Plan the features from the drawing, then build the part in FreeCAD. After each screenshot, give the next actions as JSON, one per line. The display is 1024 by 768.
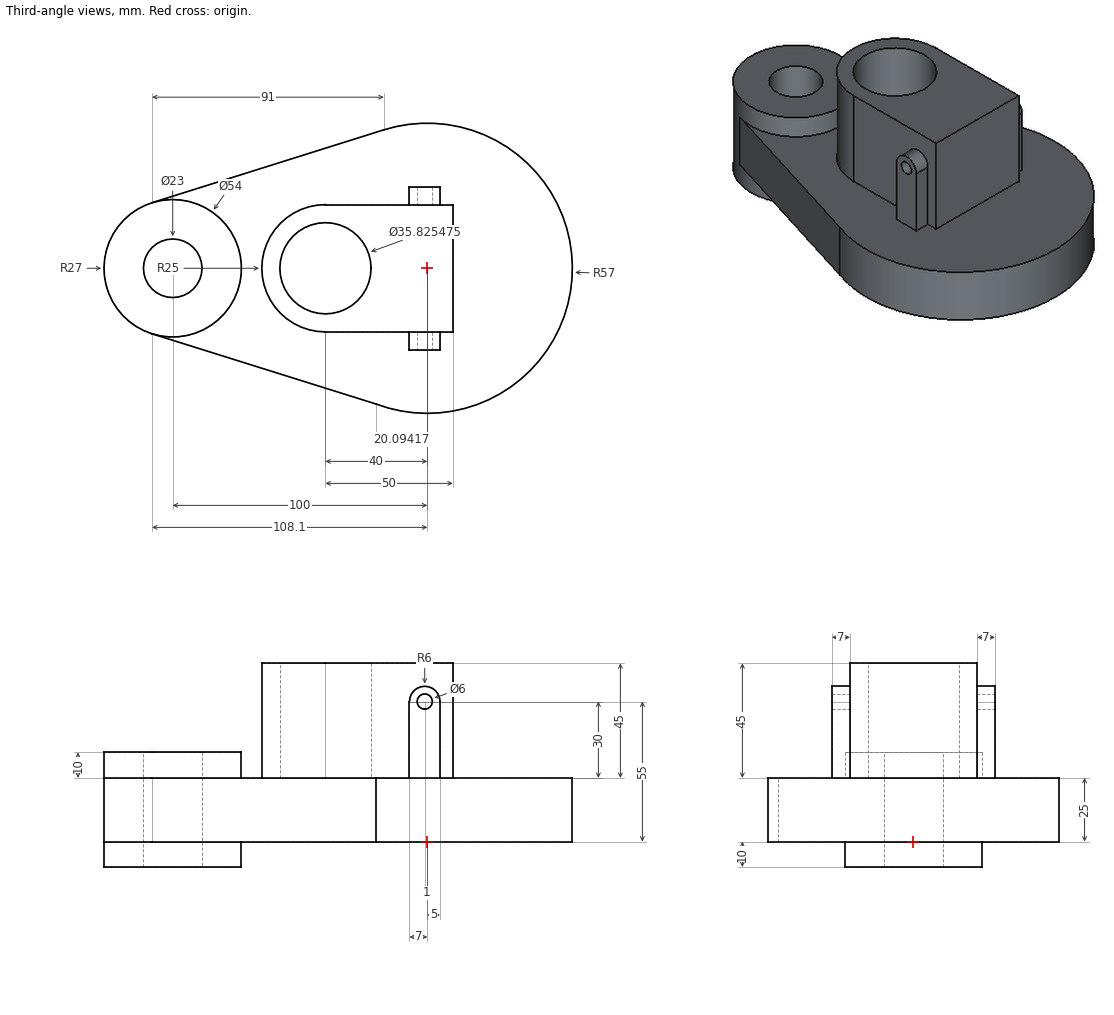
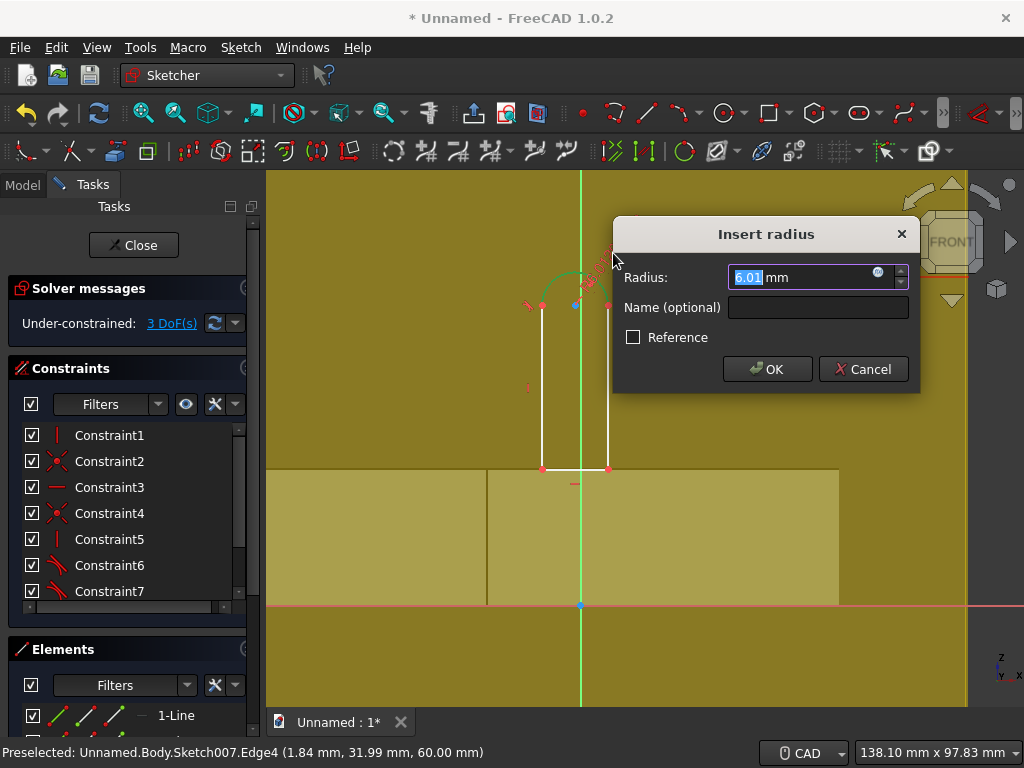
{"action": "type", "text": "6"}
{"action": "key", "text": "Return"}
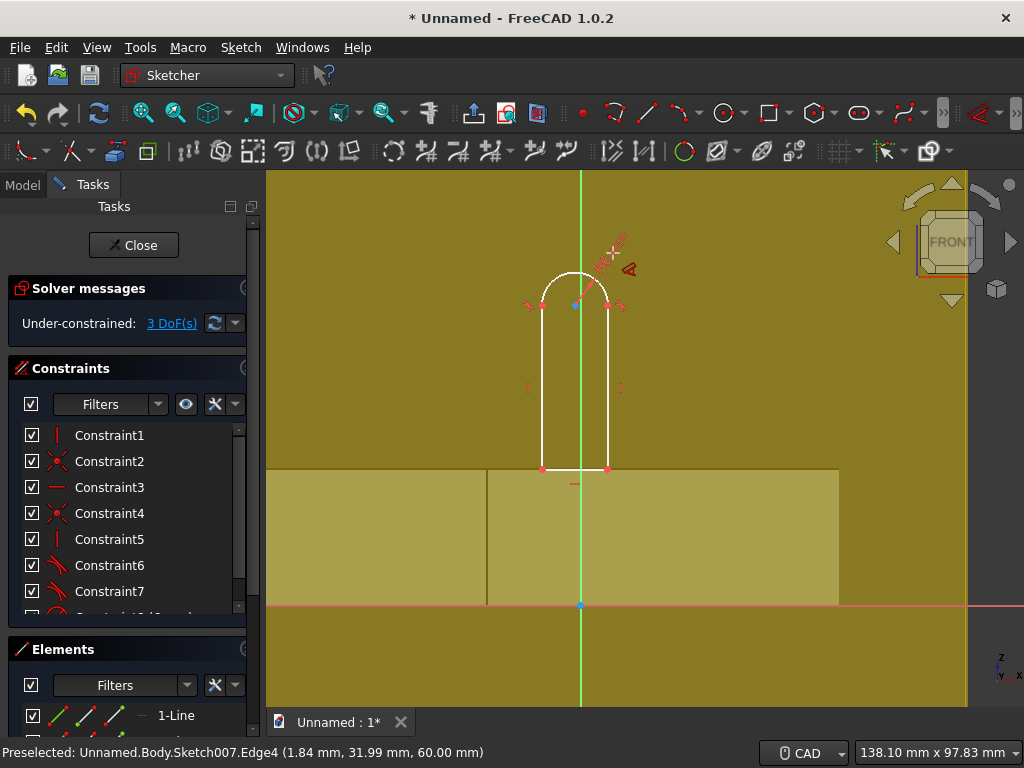
{"action": "left_click", "coordinate": [608, 355]}
{"action": "left_click", "coordinate": [642, 388]}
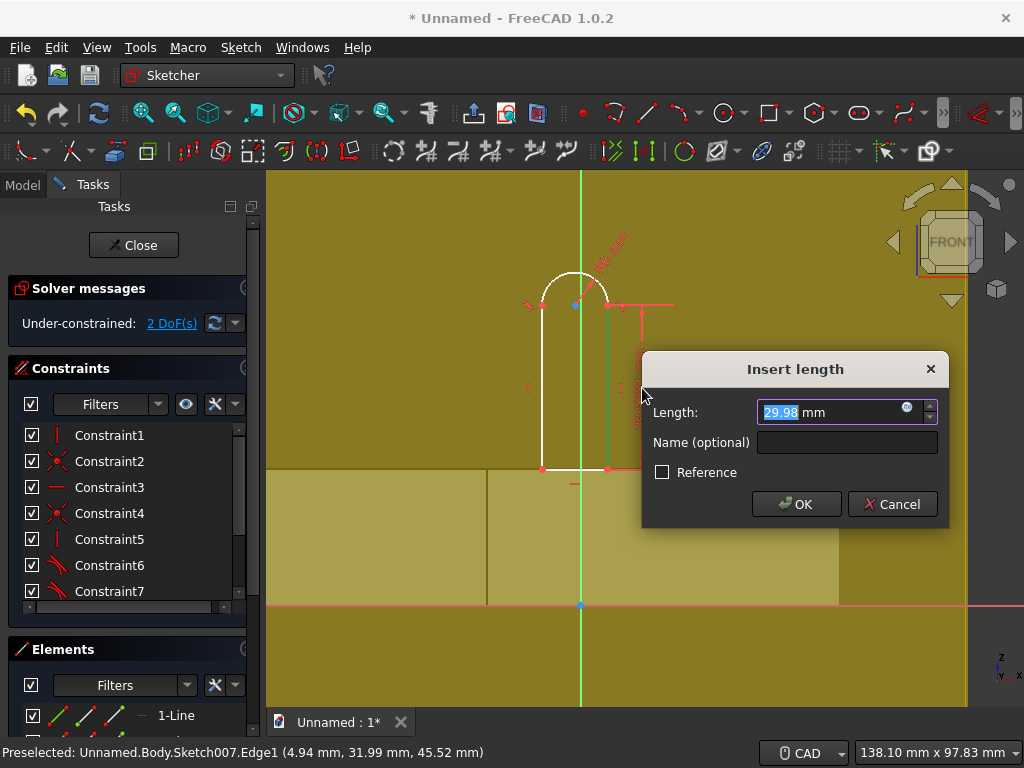
{"action": "type", "text": "30"}
{"action": "key", "text": "Return"}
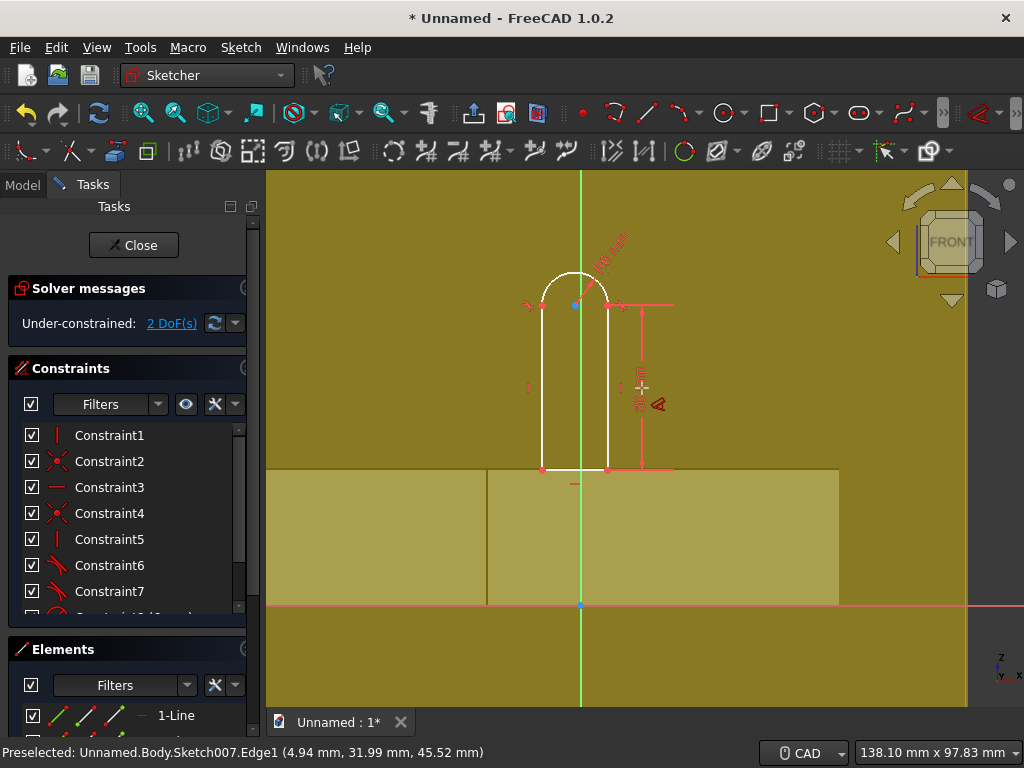
{"action": "scroll", "coordinate": [608, 305], "scroll_direction": "up", "scroll_amount": 2}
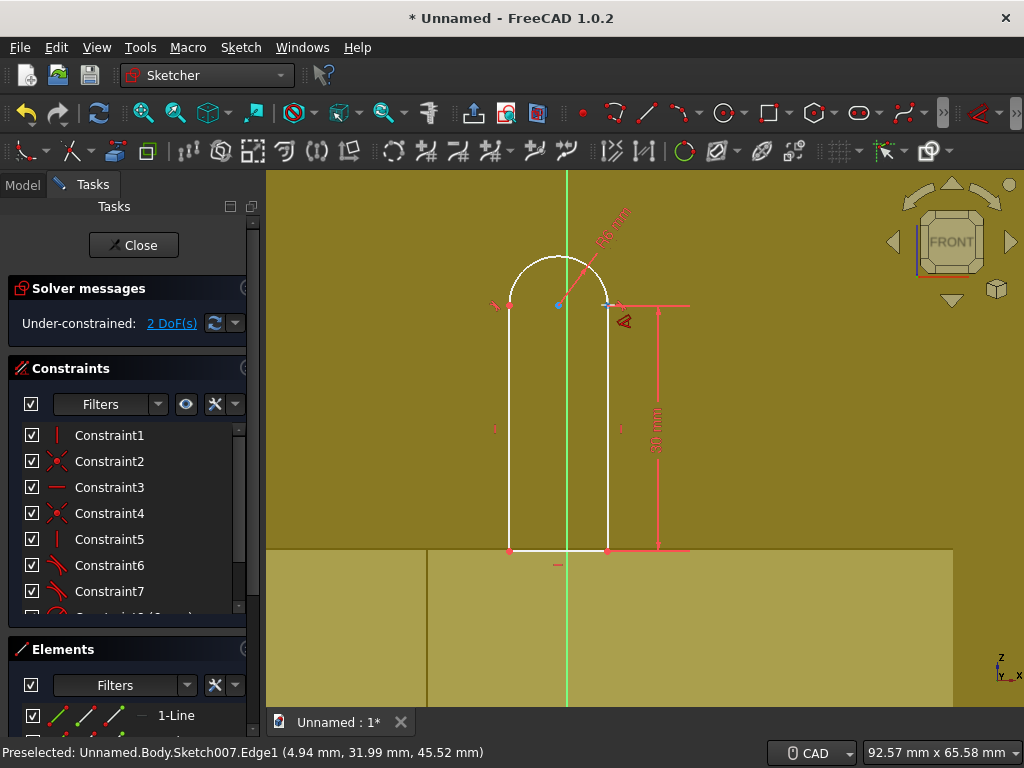
{"action": "left_click", "coordinate": [608, 306]}
{"action": "left_click", "coordinate": [587, 248]}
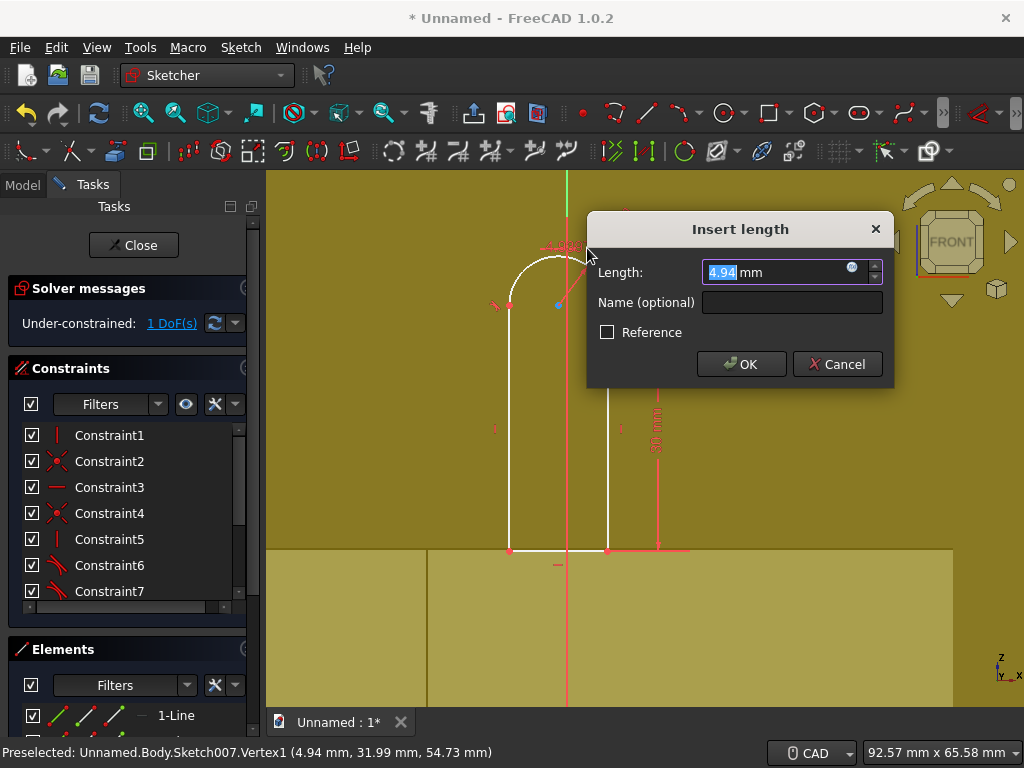
{"action": "type", "text": "5"}
{"action": "key", "text": "Return"}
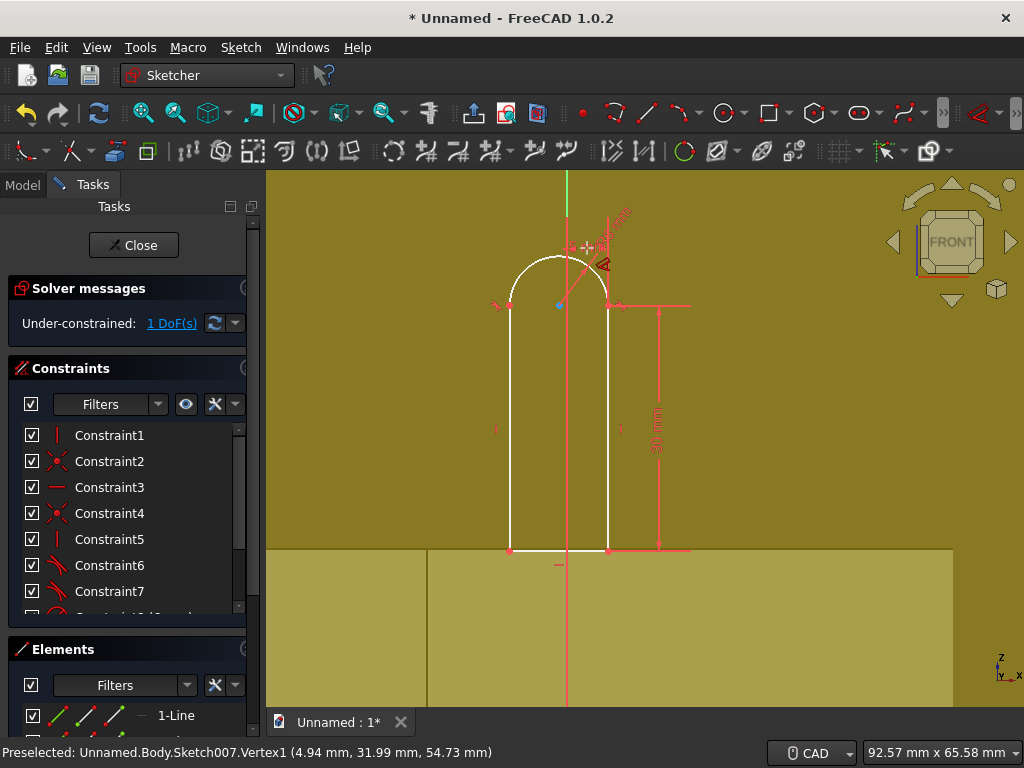
{"action": "left_click", "coordinate": [608, 306]}
{"action": "left_click", "coordinate": [642, 492]}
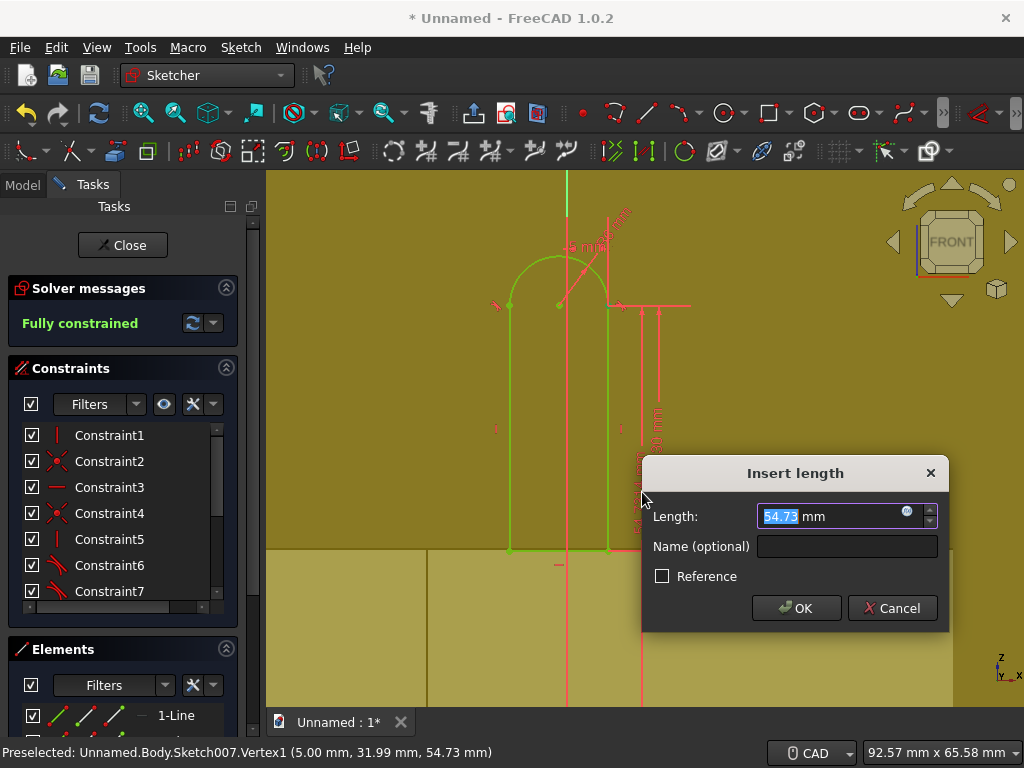
{"action": "type", "text": "55"}
{"action": "key", "text": "Return"}
{"action": "key", "text": "Escape"}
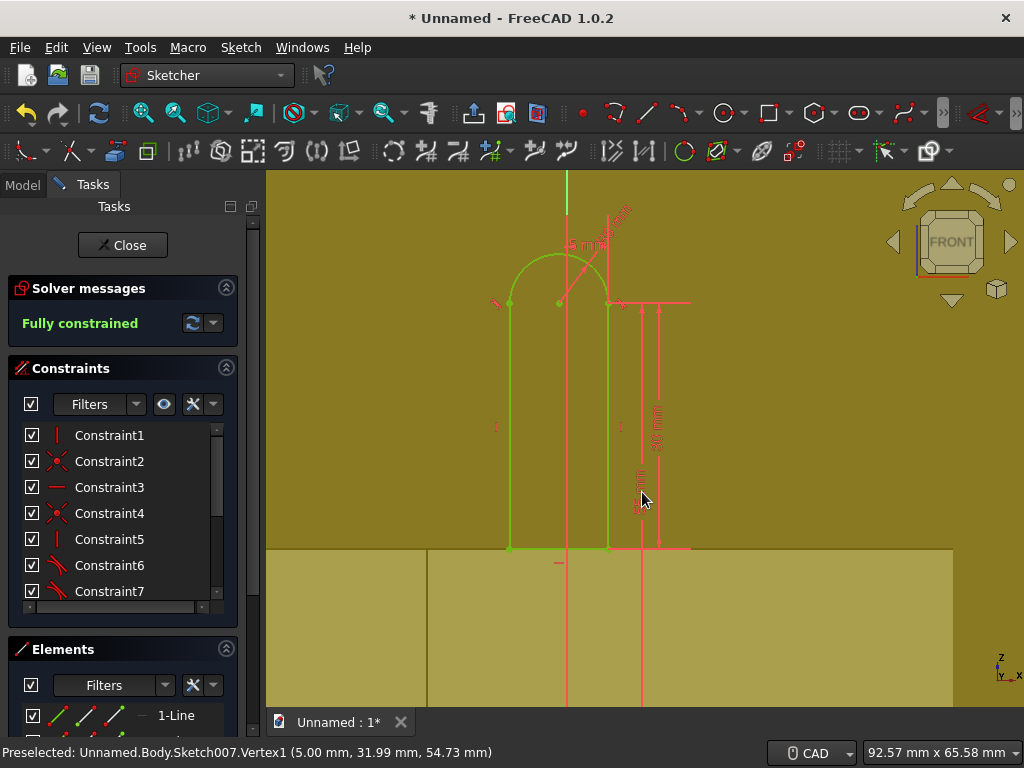
{"action": "left_click", "coordinate": [123, 245]}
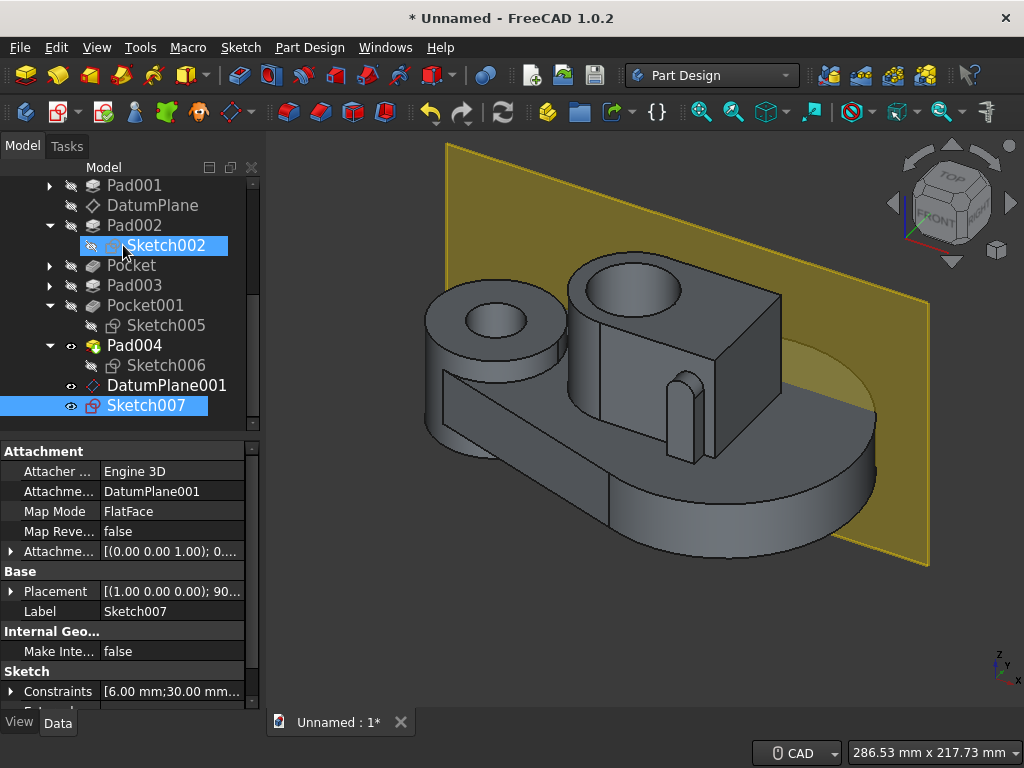
{"action": "left_click", "coordinate": [26, 76]}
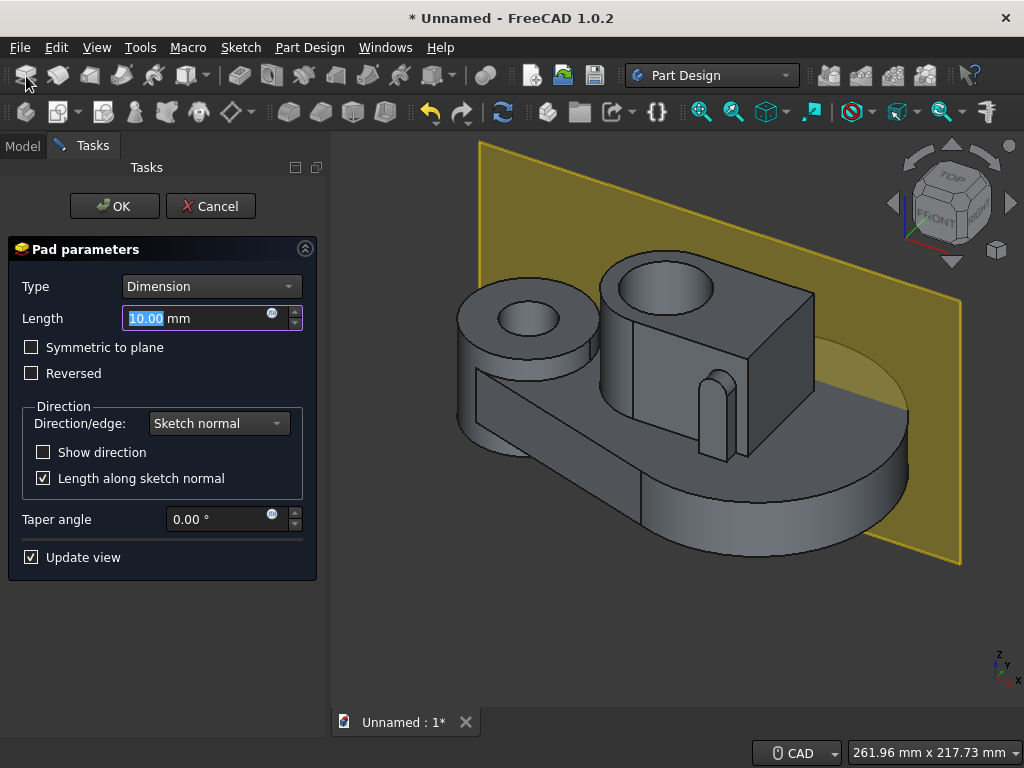
{"action": "type", "text": "7"}
{"action": "key", "text": "Tab"}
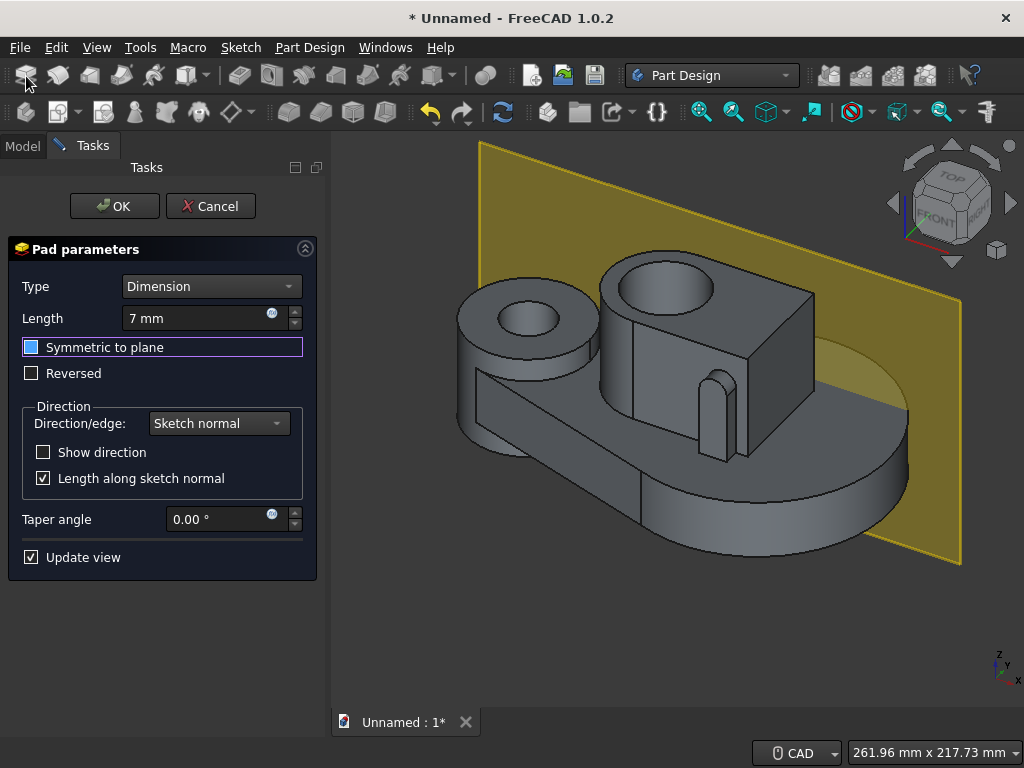
{"action": "left_click", "coordinate": [115, 206]}